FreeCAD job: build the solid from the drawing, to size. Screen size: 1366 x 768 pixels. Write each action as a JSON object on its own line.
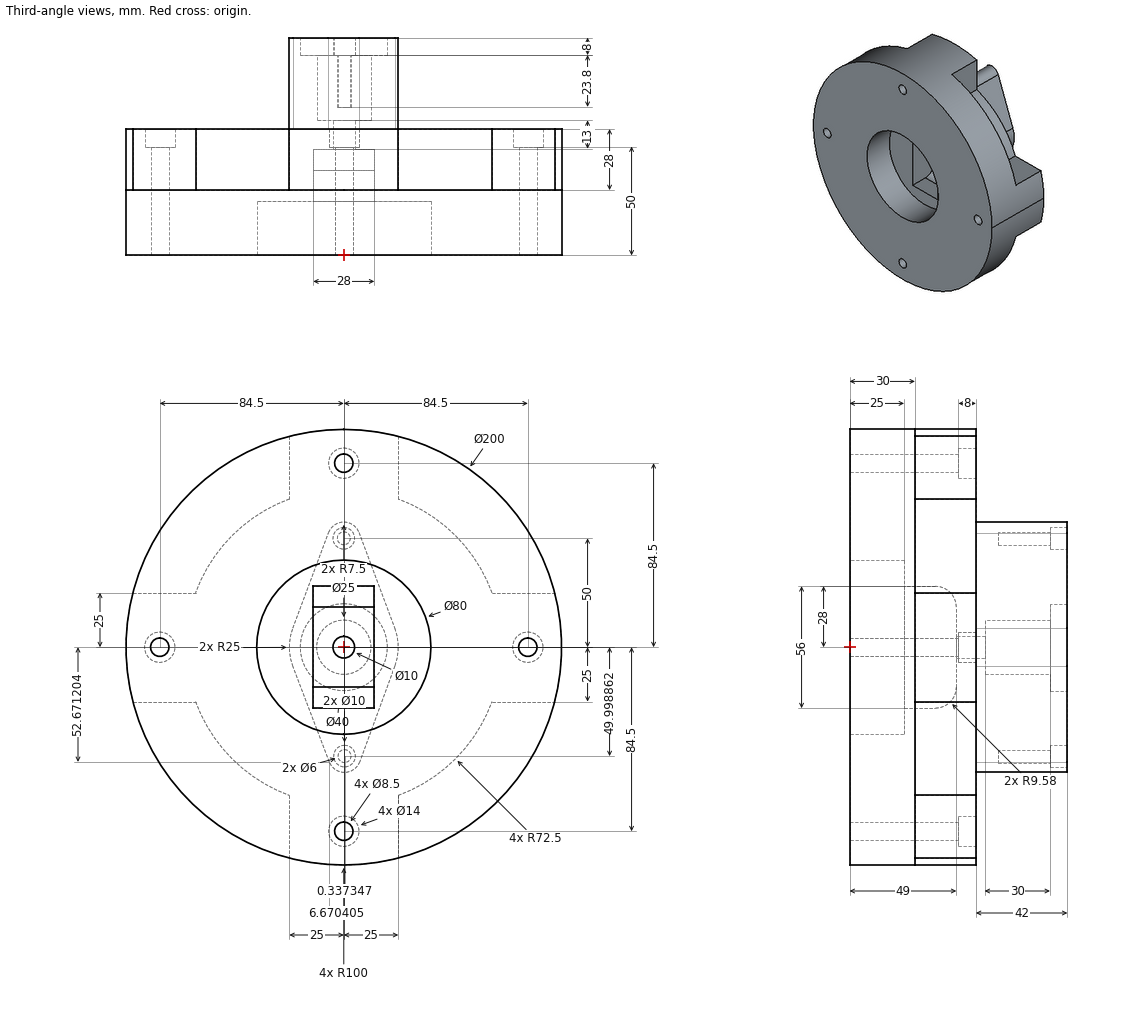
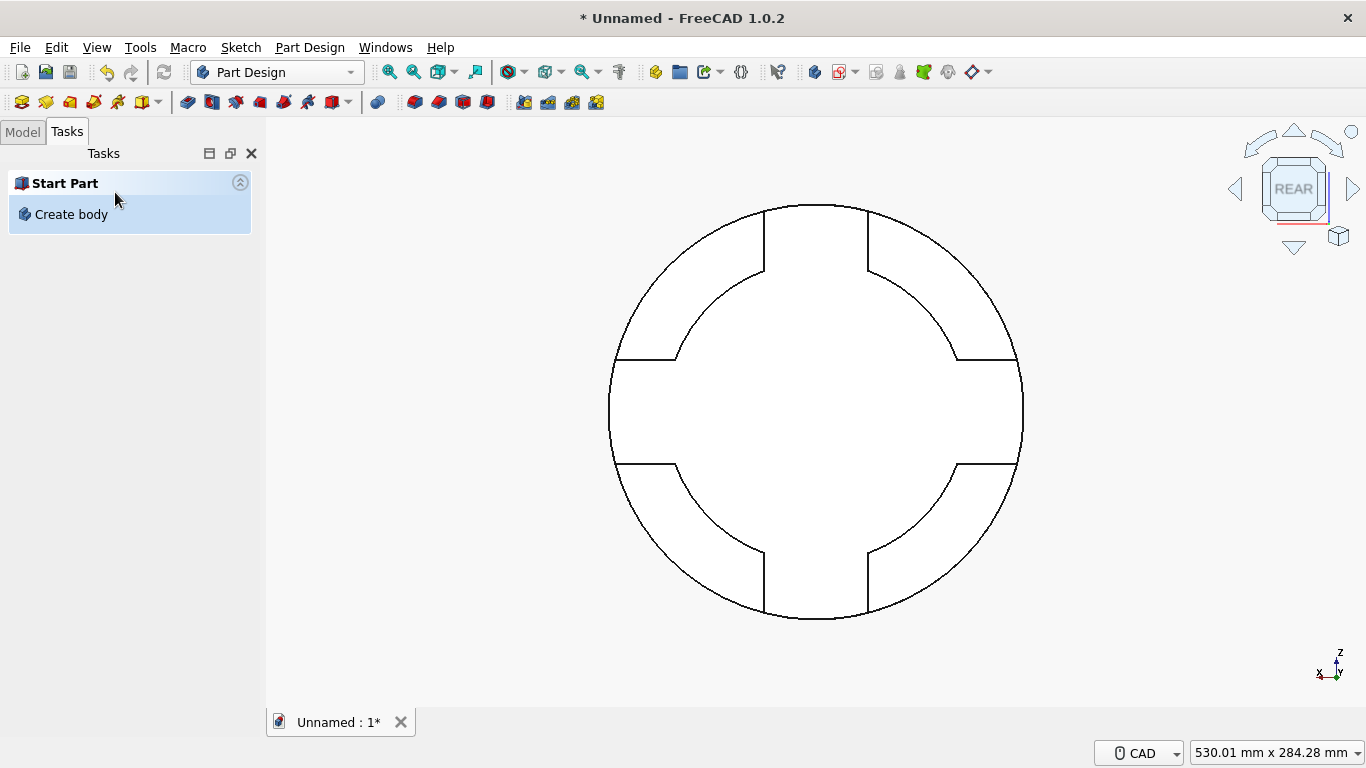
{"action": "left_click", "coordinate": [816, 411]}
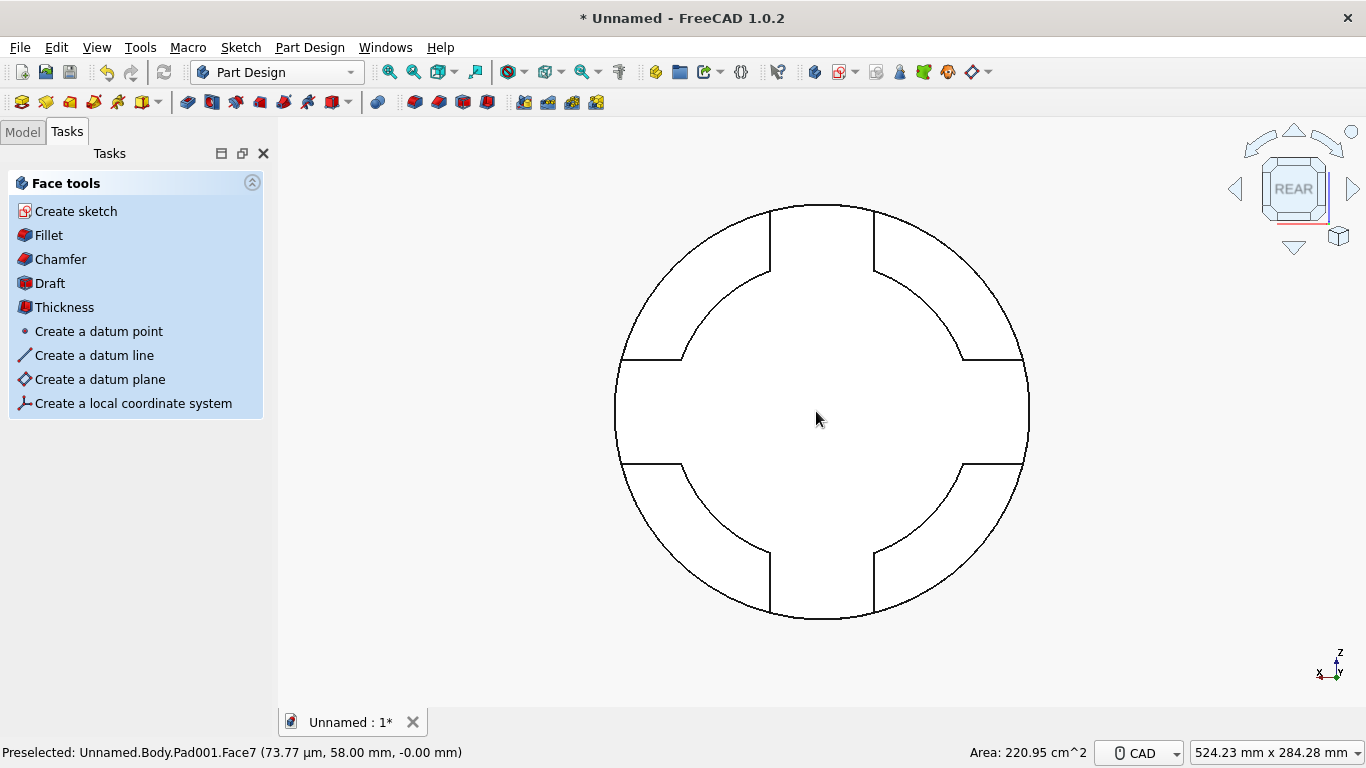
{"action": "left_click", "coordinate": [840, 72]}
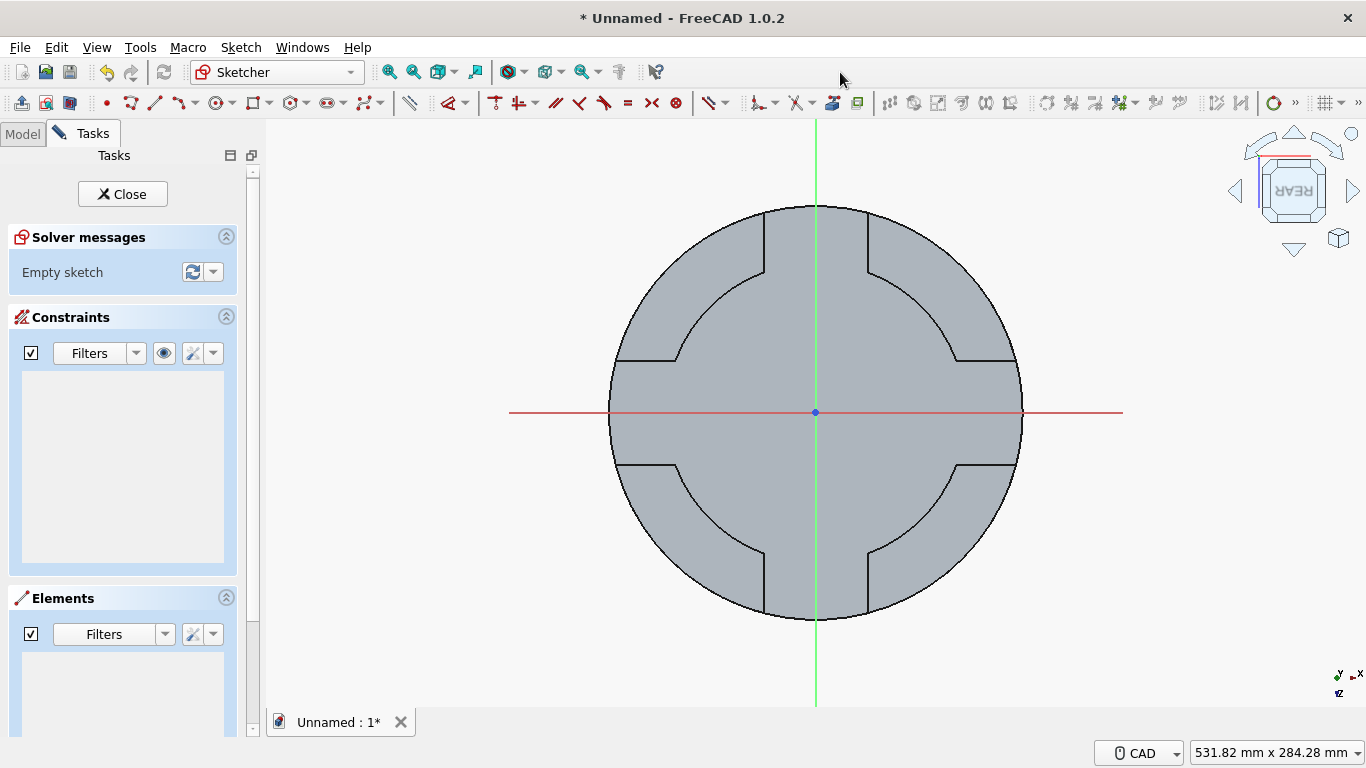
{"action": "left_click", "coordinate": [216, 104]}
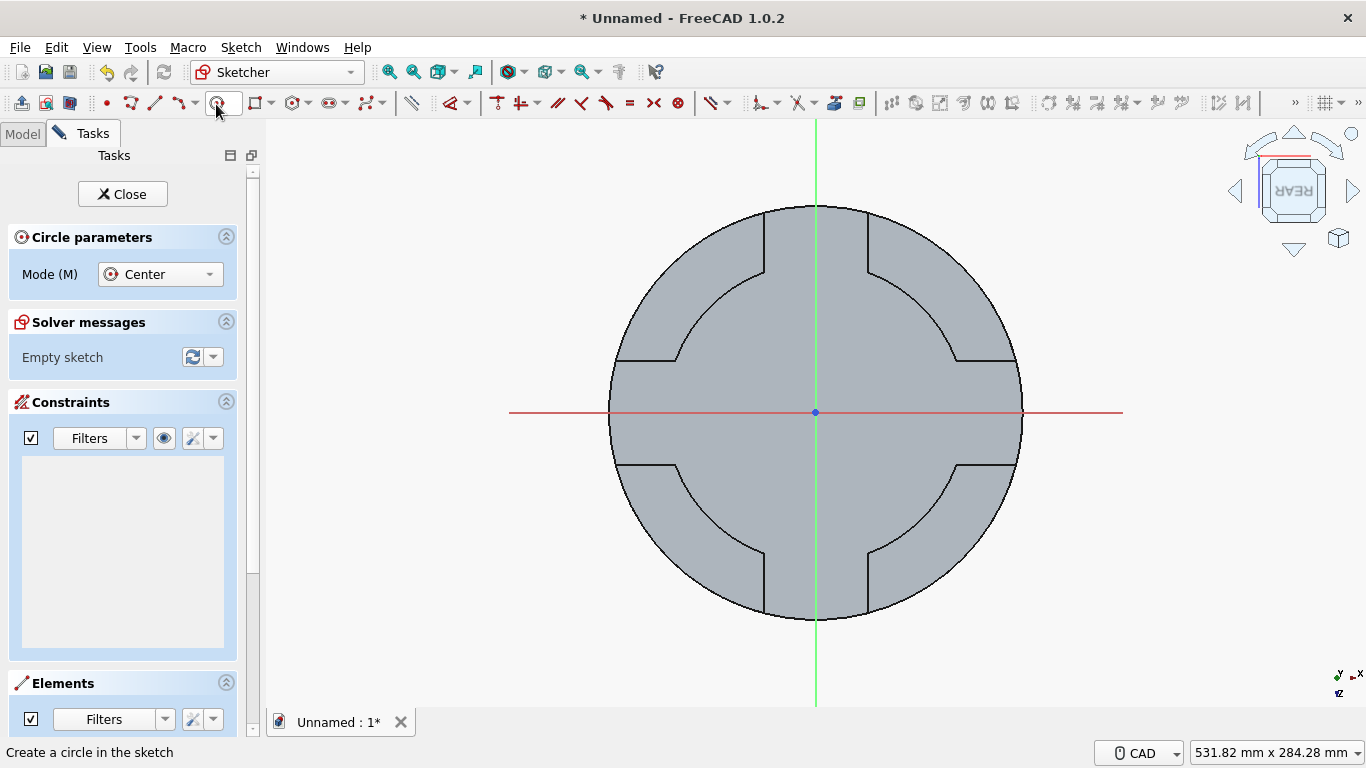
{"action": "scroll", "coordinate": [816, 238], "scroll_direction": "up", "scroll_amount": 3}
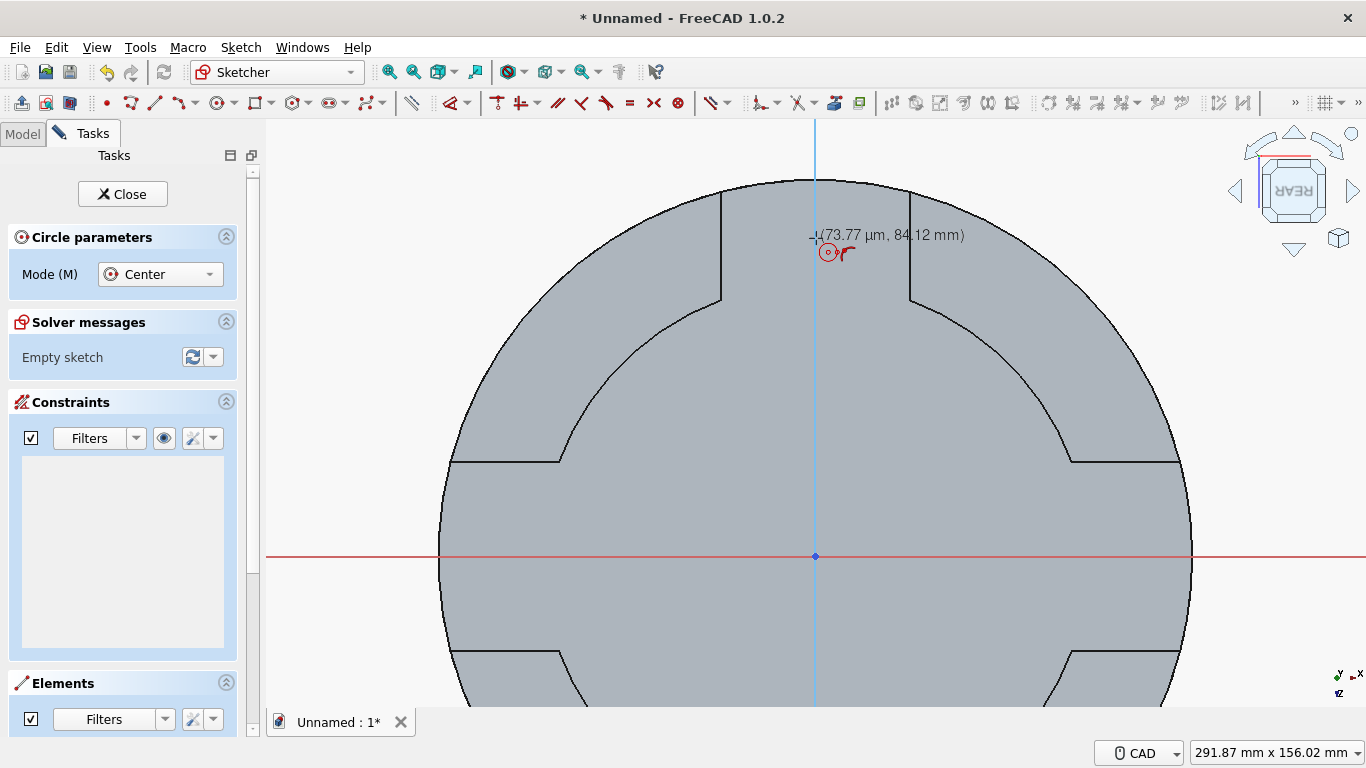
{"action": "left_click", "coordinate": [815, 238]}
{"action": "left_click", "coordinate": [834, 220]}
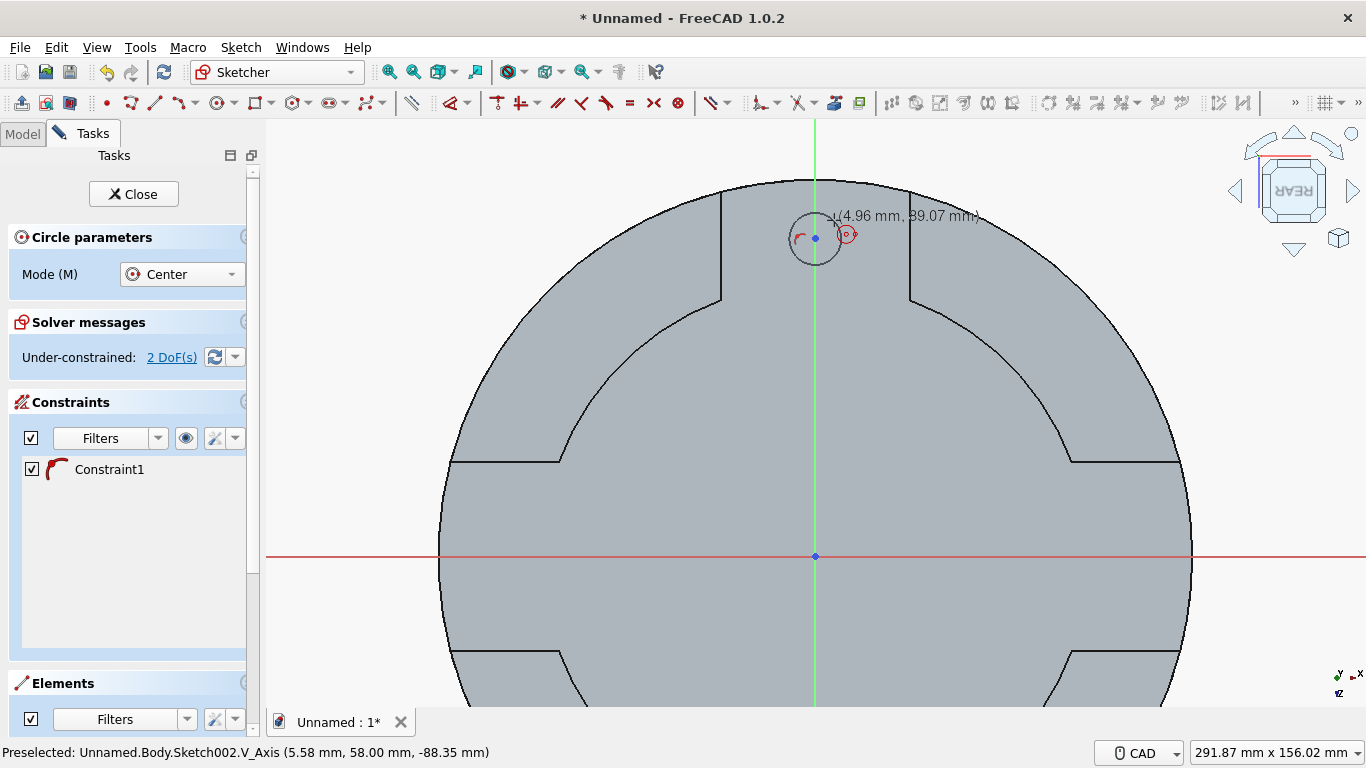
{"action": "left_click", "coordinate": [1134, 557]}
{"action": "left_click", "coordinate": [1152, 538]}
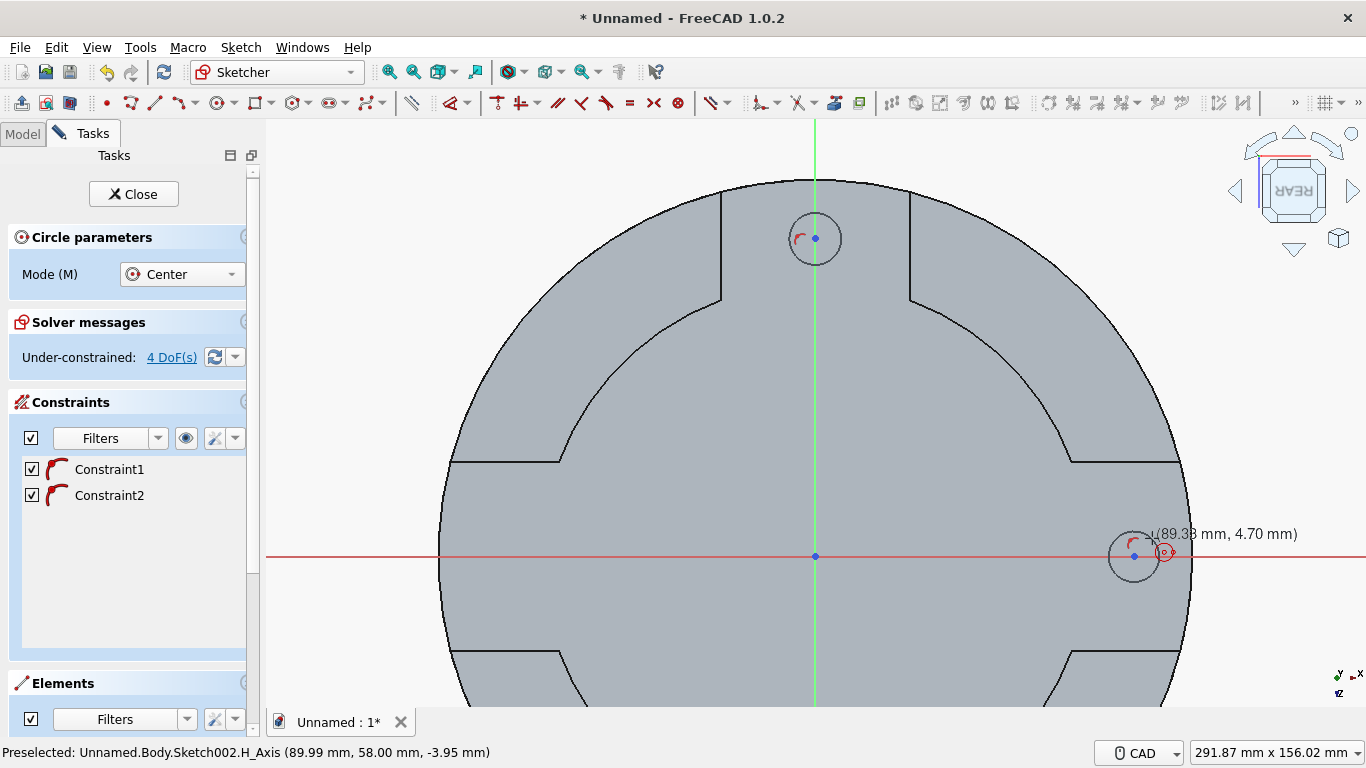
{"action": "scroll", "coordinate": [665, 238], "scroll_direction": "down", "scroll_amount": 3}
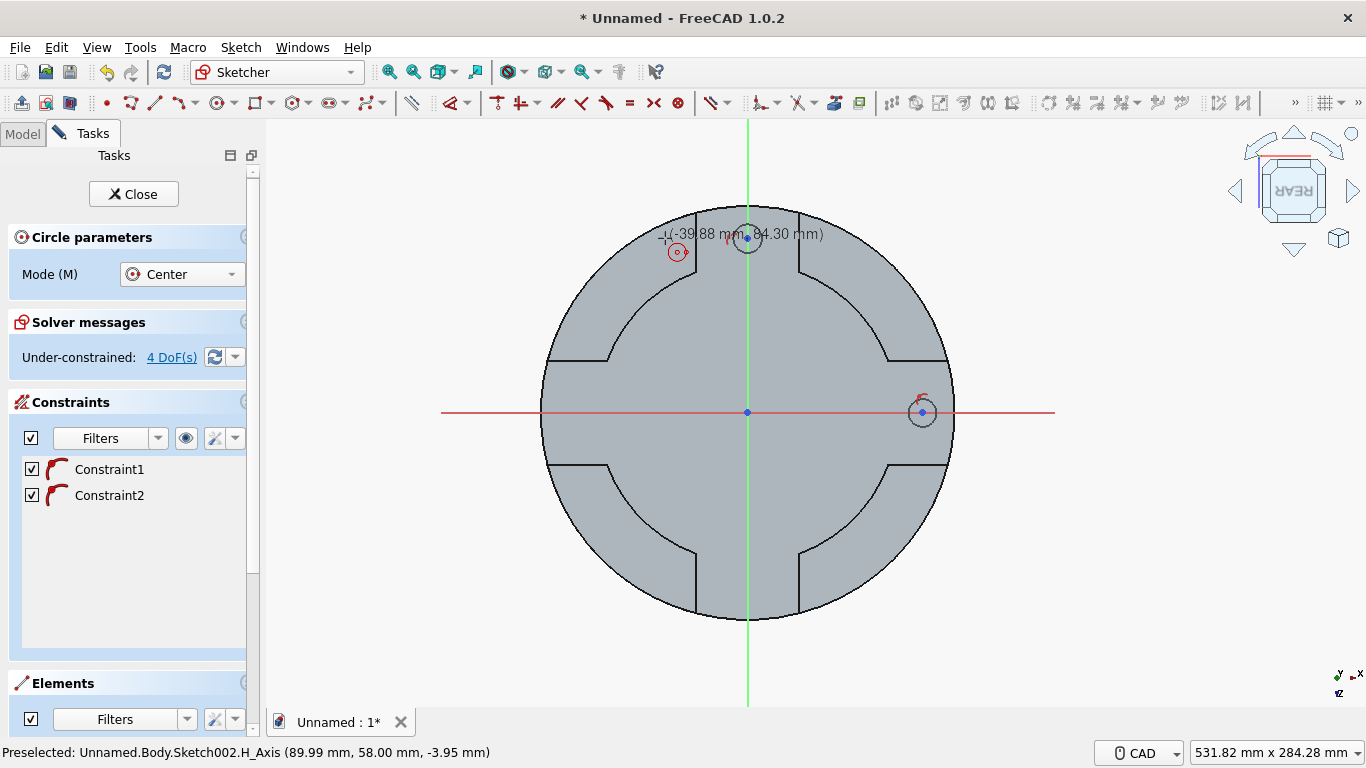
{"action": "scroll", "coordinate": [748, 588], "scroll_direction": "up", "scroll_amount": 3}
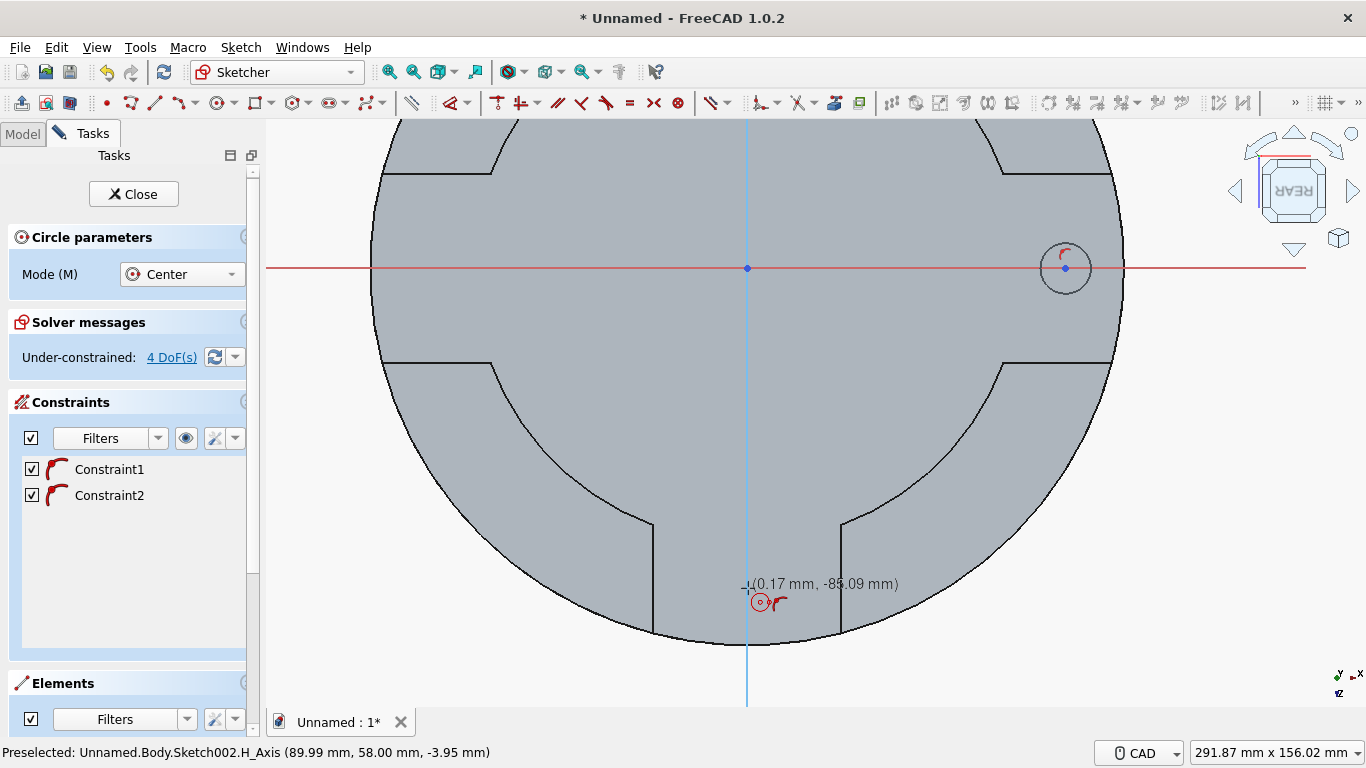
{"action": "left_click", "coordinate": [747, 587]}
{"action": "left_click", "coordinate": [766, 568]}